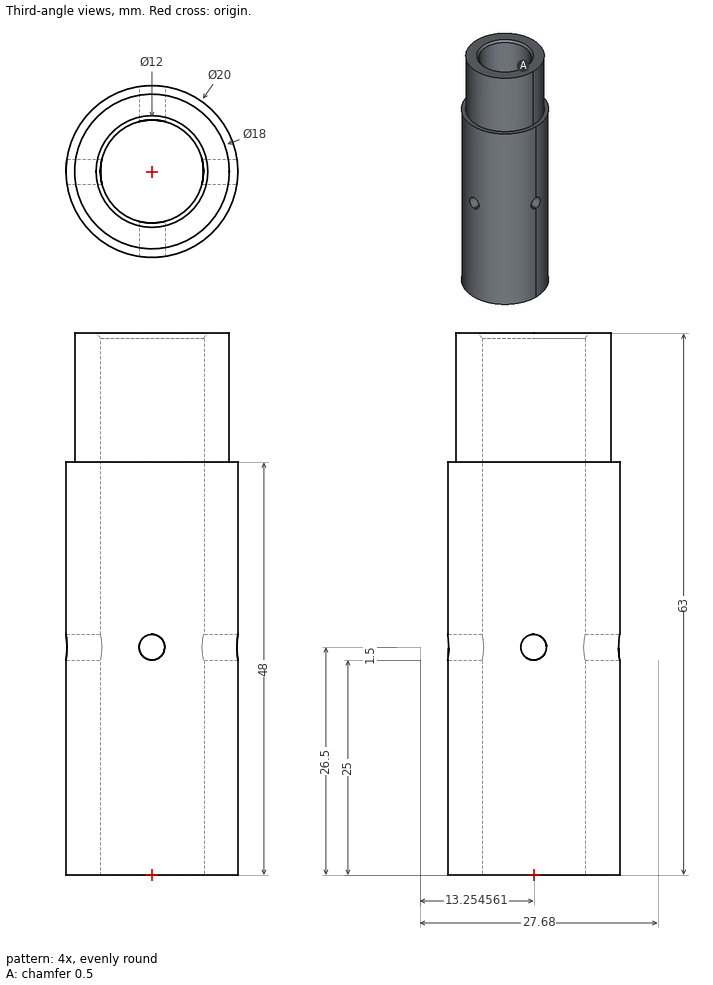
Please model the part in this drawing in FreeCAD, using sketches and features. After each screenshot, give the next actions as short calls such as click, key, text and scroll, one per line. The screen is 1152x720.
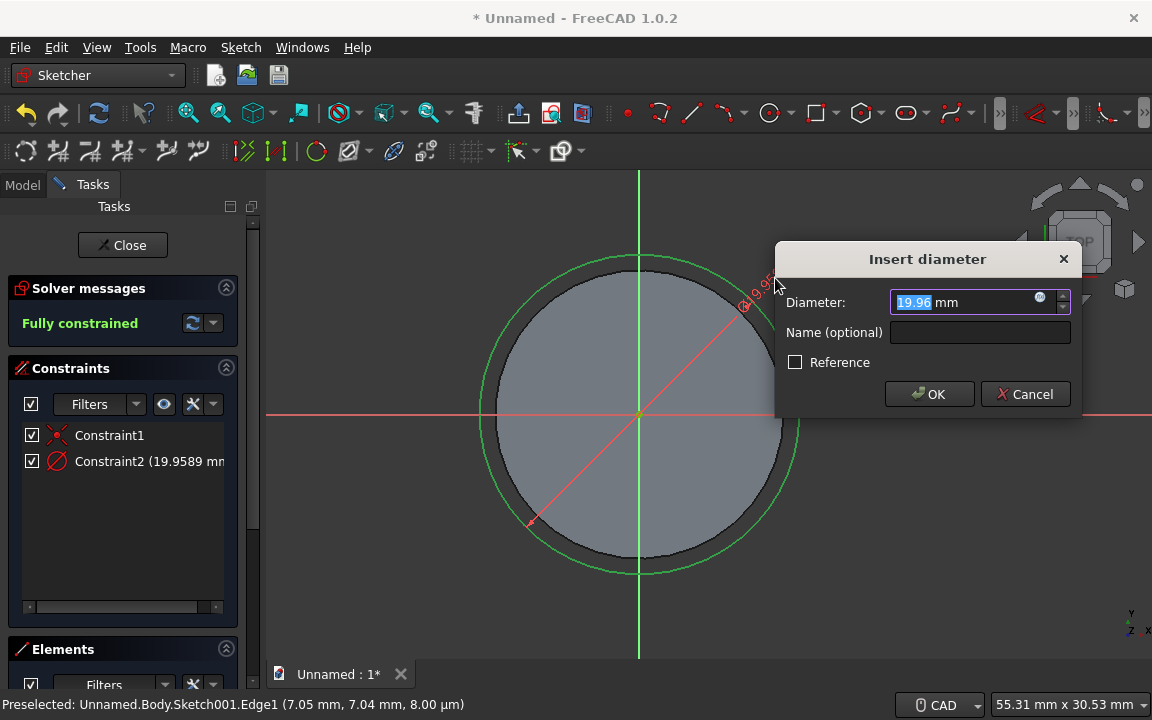
text(20)
key(Return)
key(Escape)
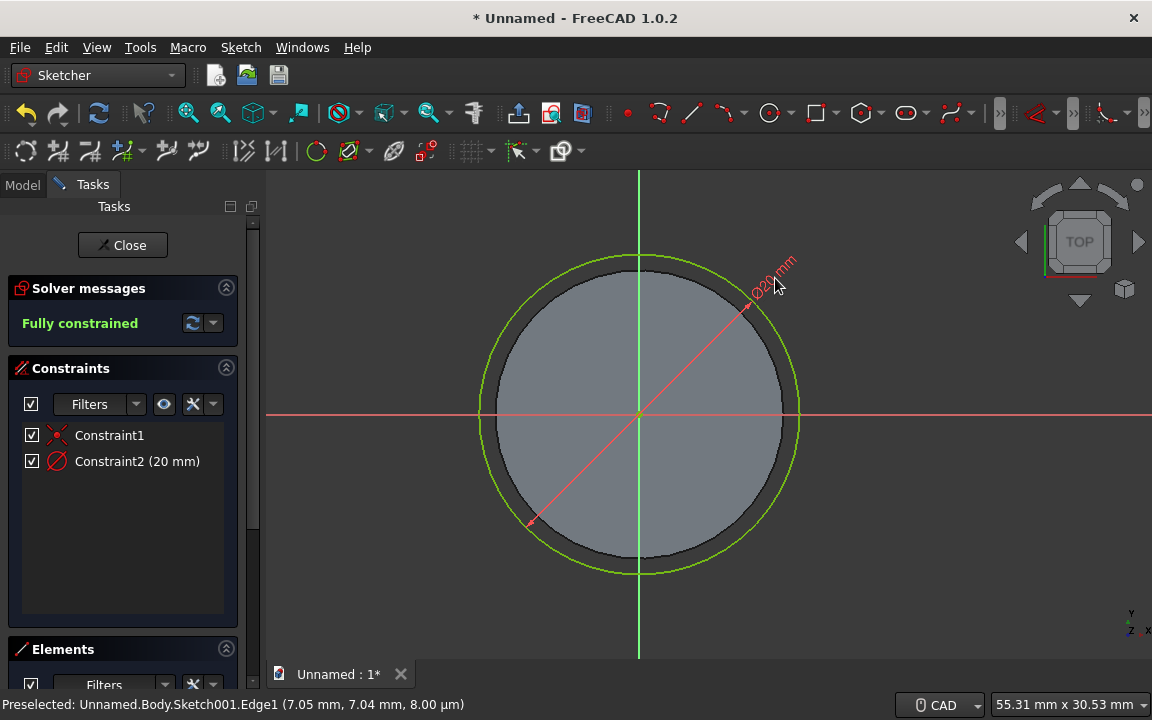
click(123, 245)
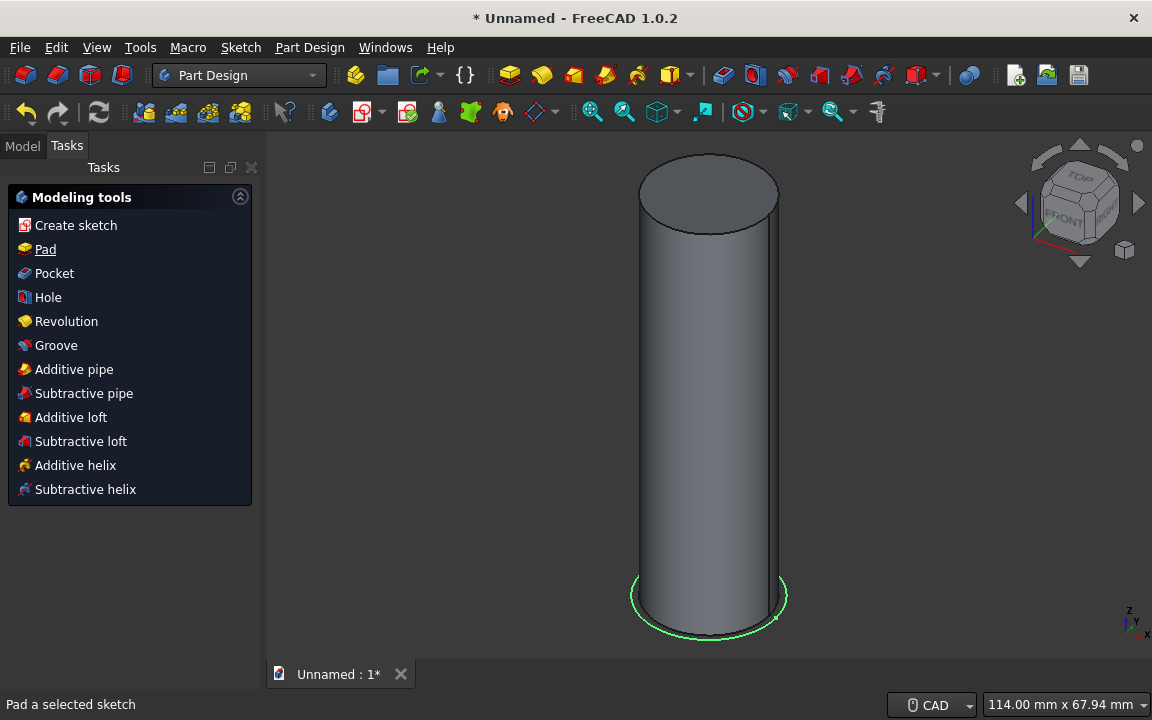
click(510, 76)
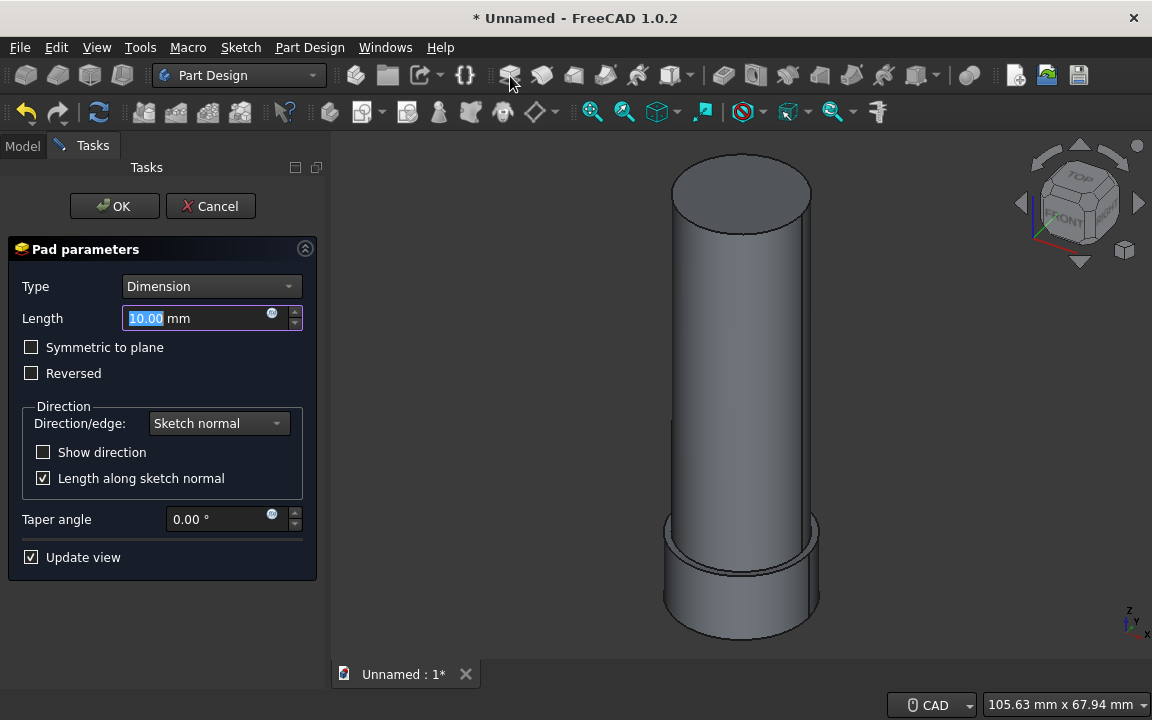
text(48)
key(Tab)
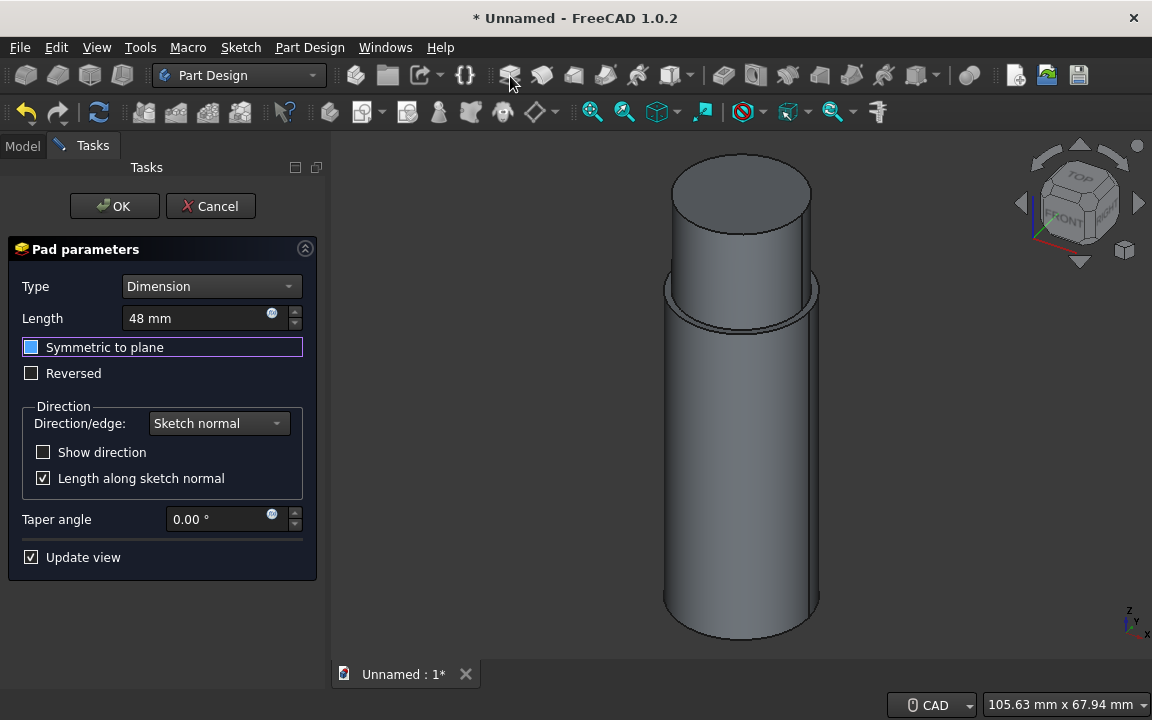
click(115, 206)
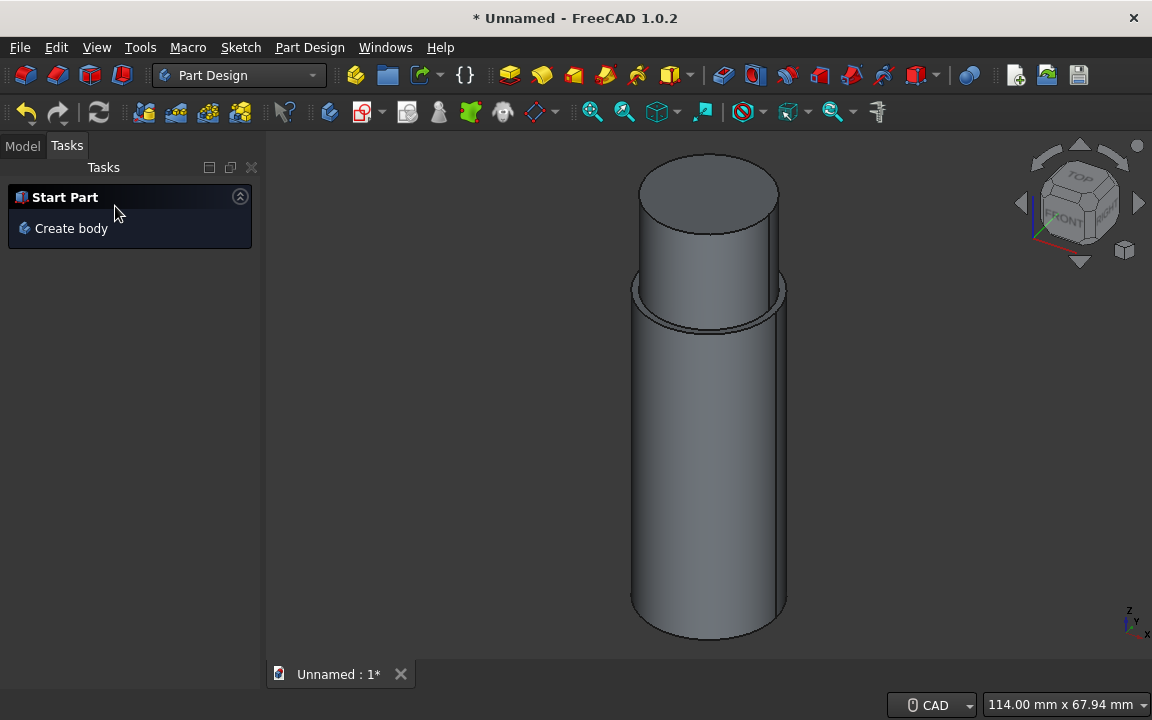
key(5)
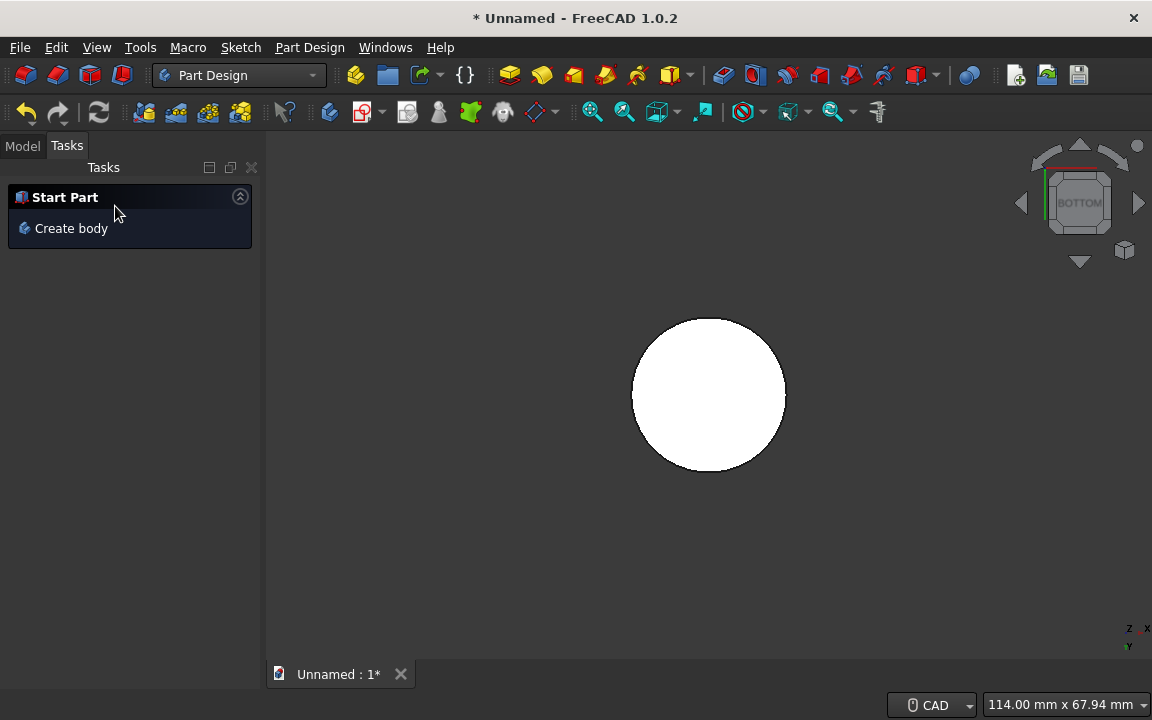
click(594, 112)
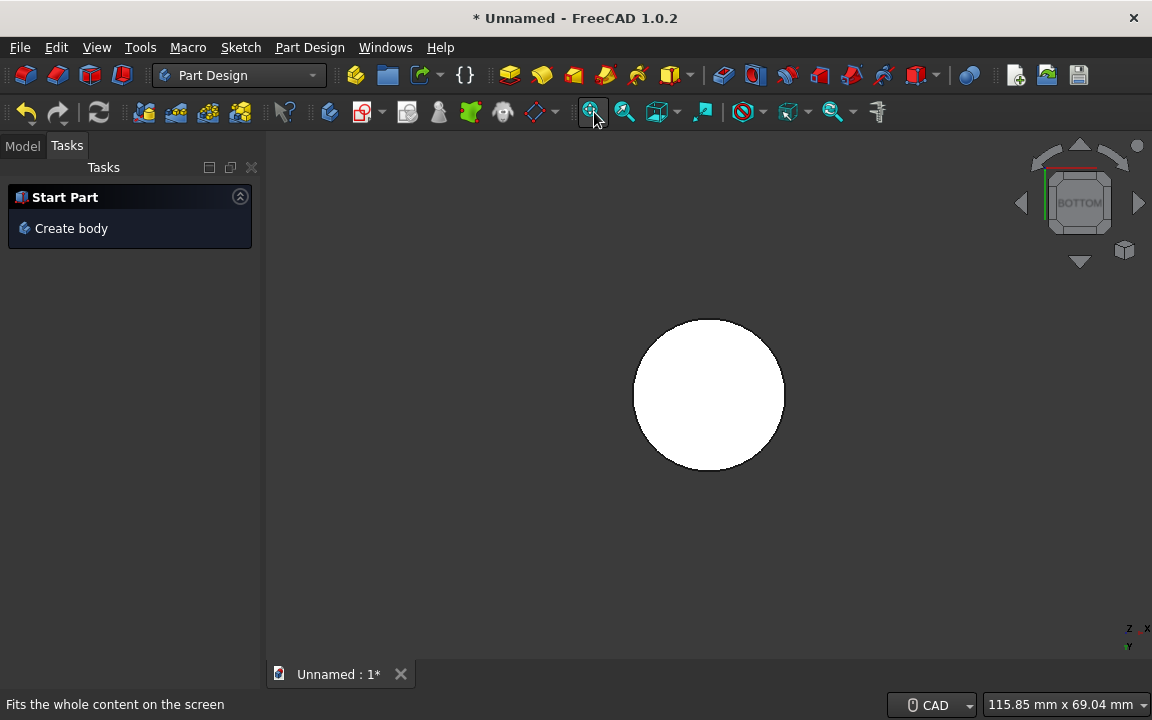
click(709, 394)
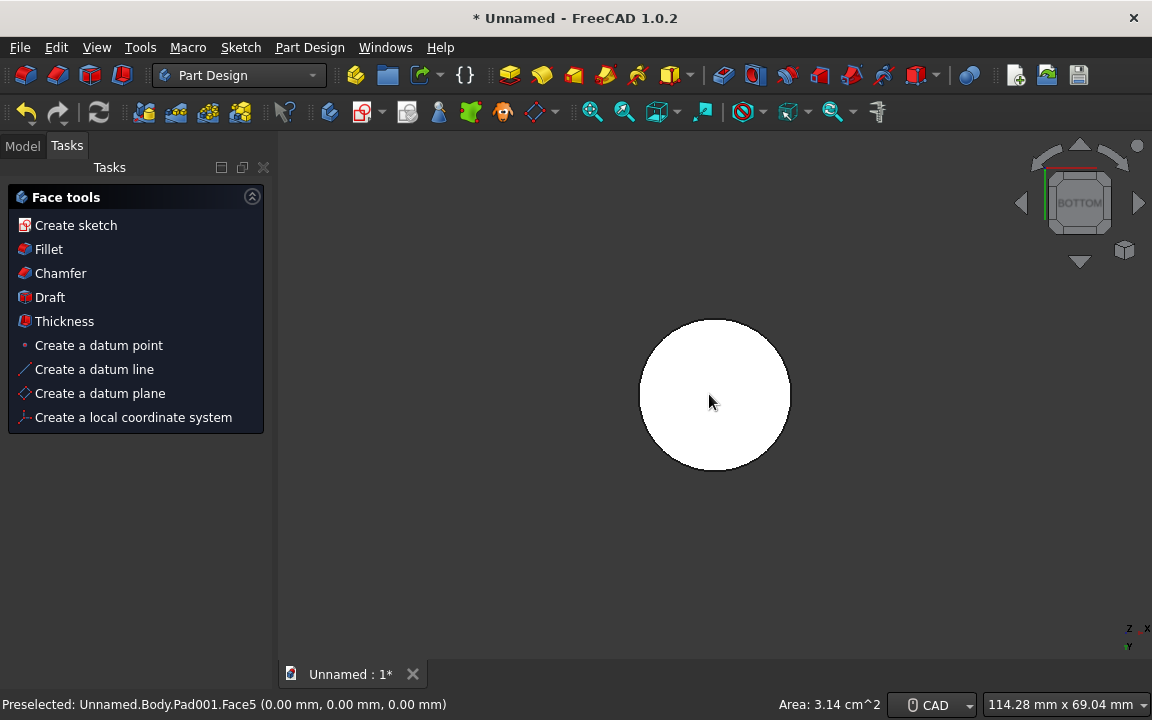
click(362, 112)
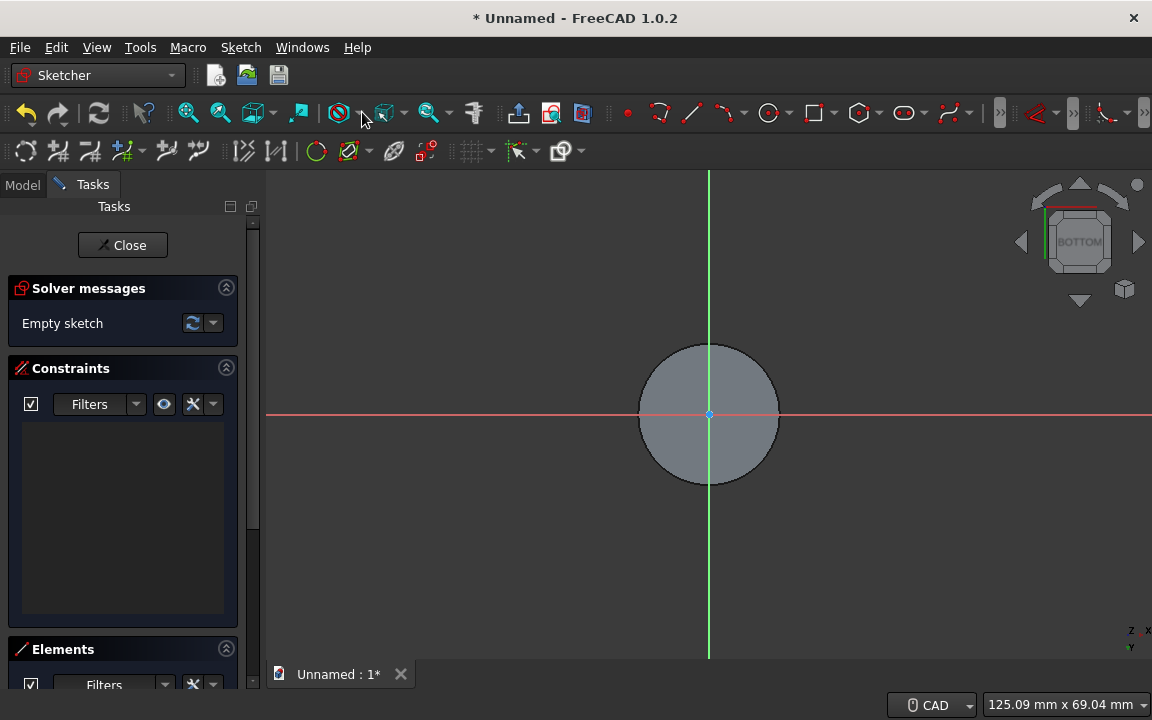
scroll(739, 415, up, 6)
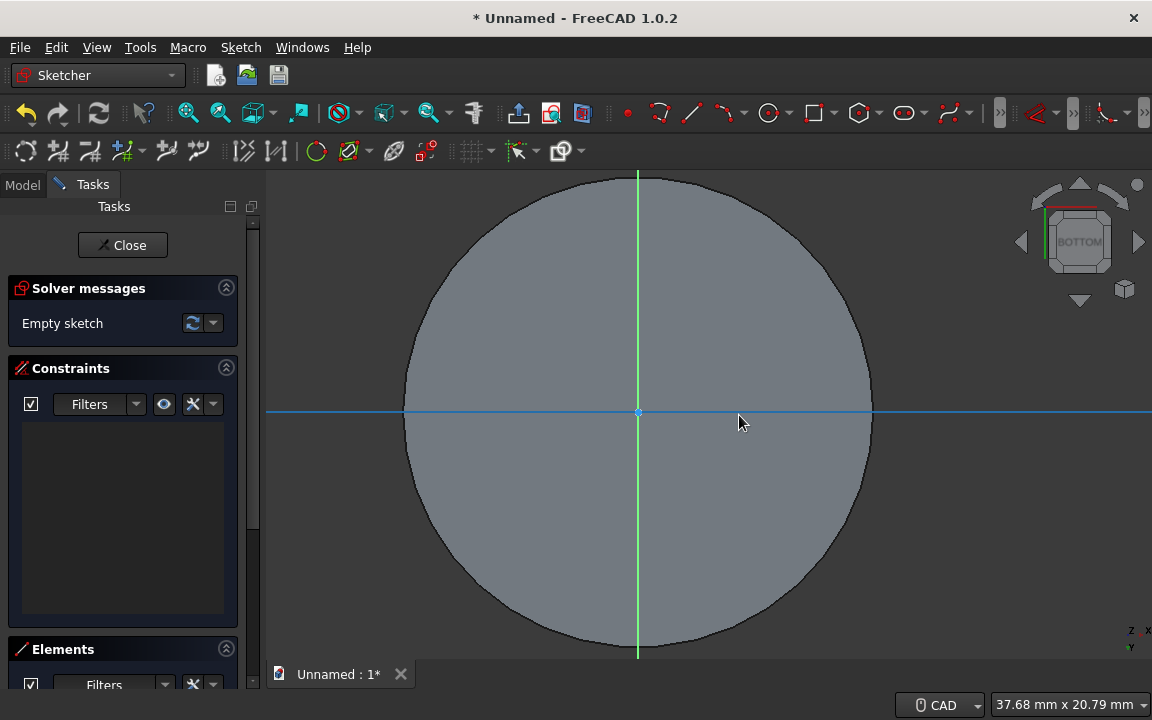
click(770, 114)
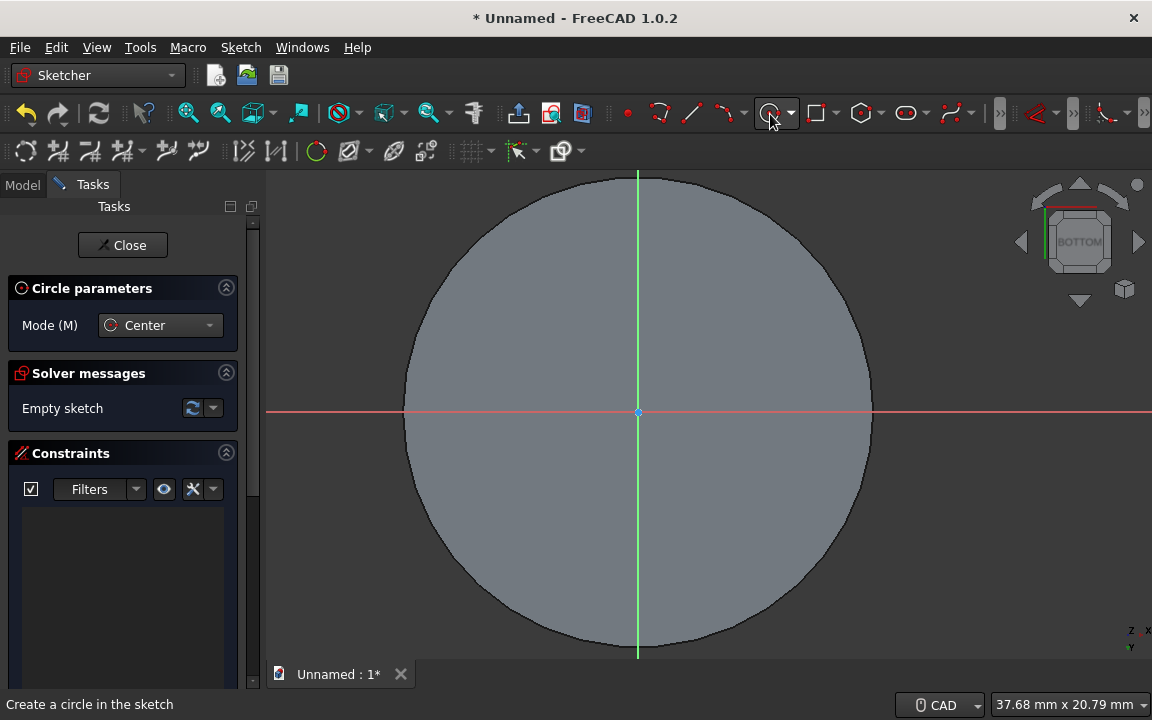
click(638, 412)
click(738, 312)
key(Escape)